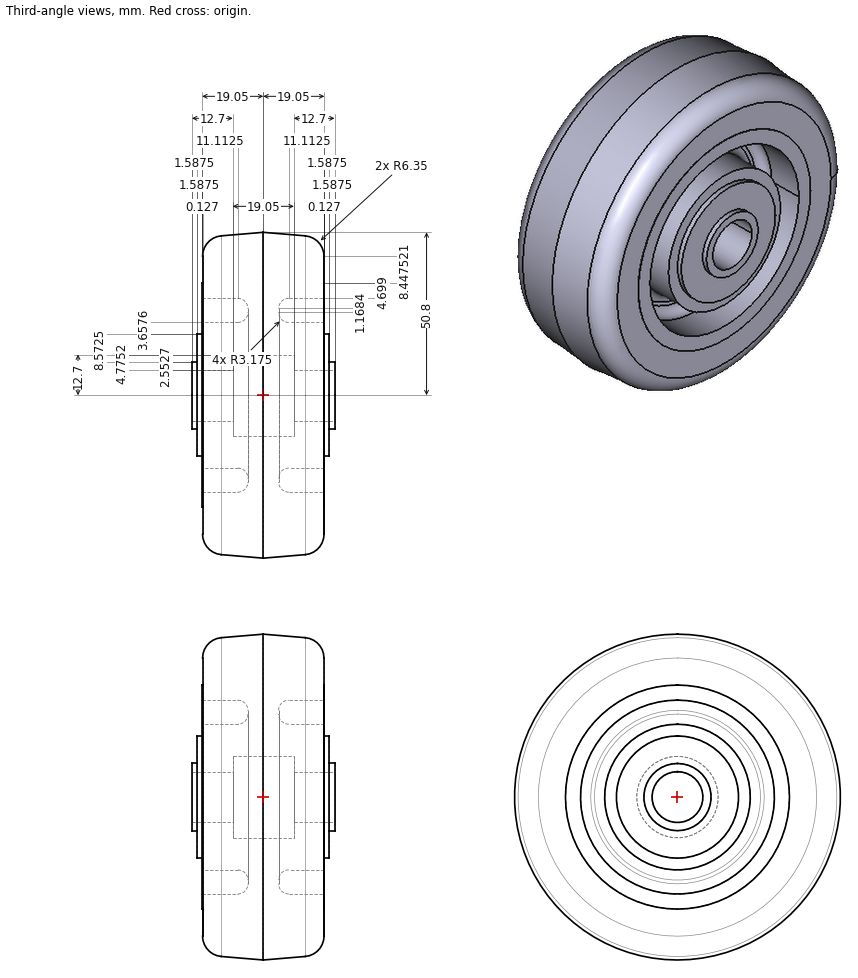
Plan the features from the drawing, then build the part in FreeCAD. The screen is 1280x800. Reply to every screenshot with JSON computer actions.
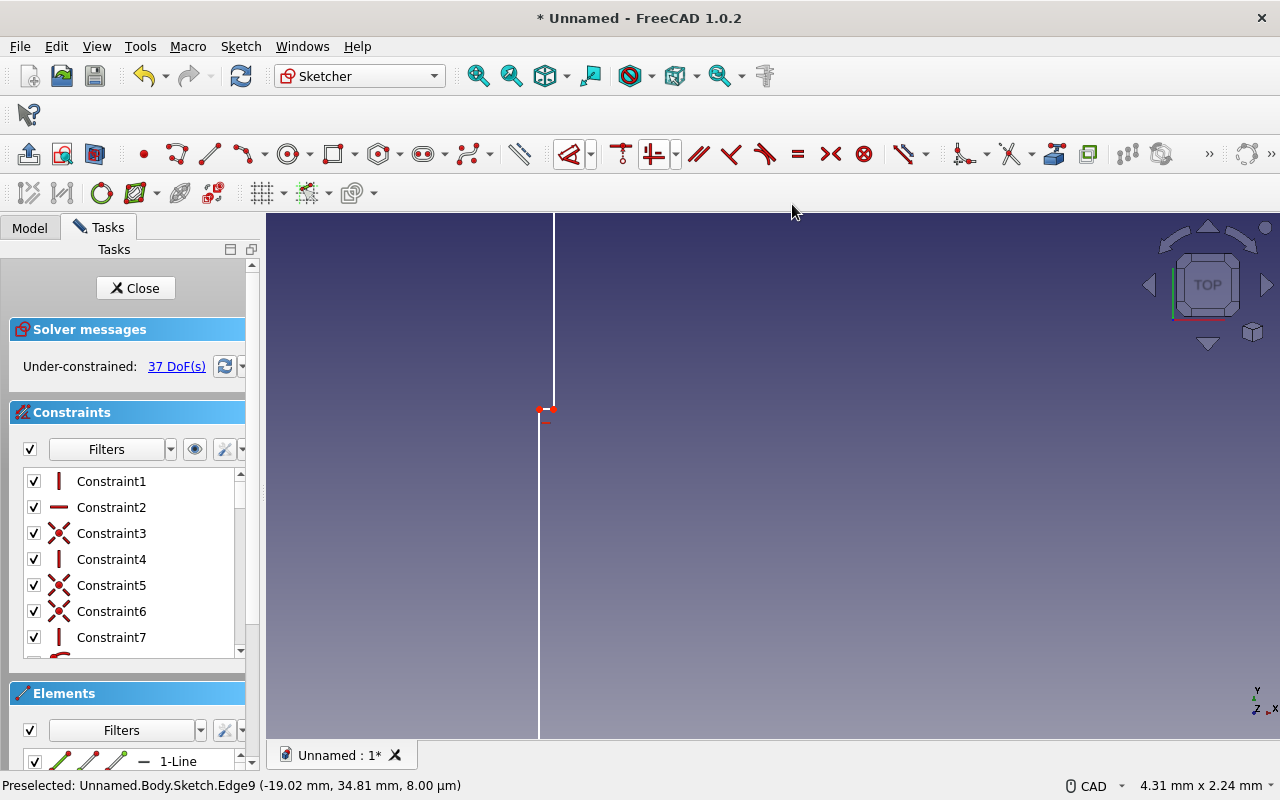
{"action": "scroll", "coordinate": [556, 402], "scroll_direction": "down", "scroll_amount": 17}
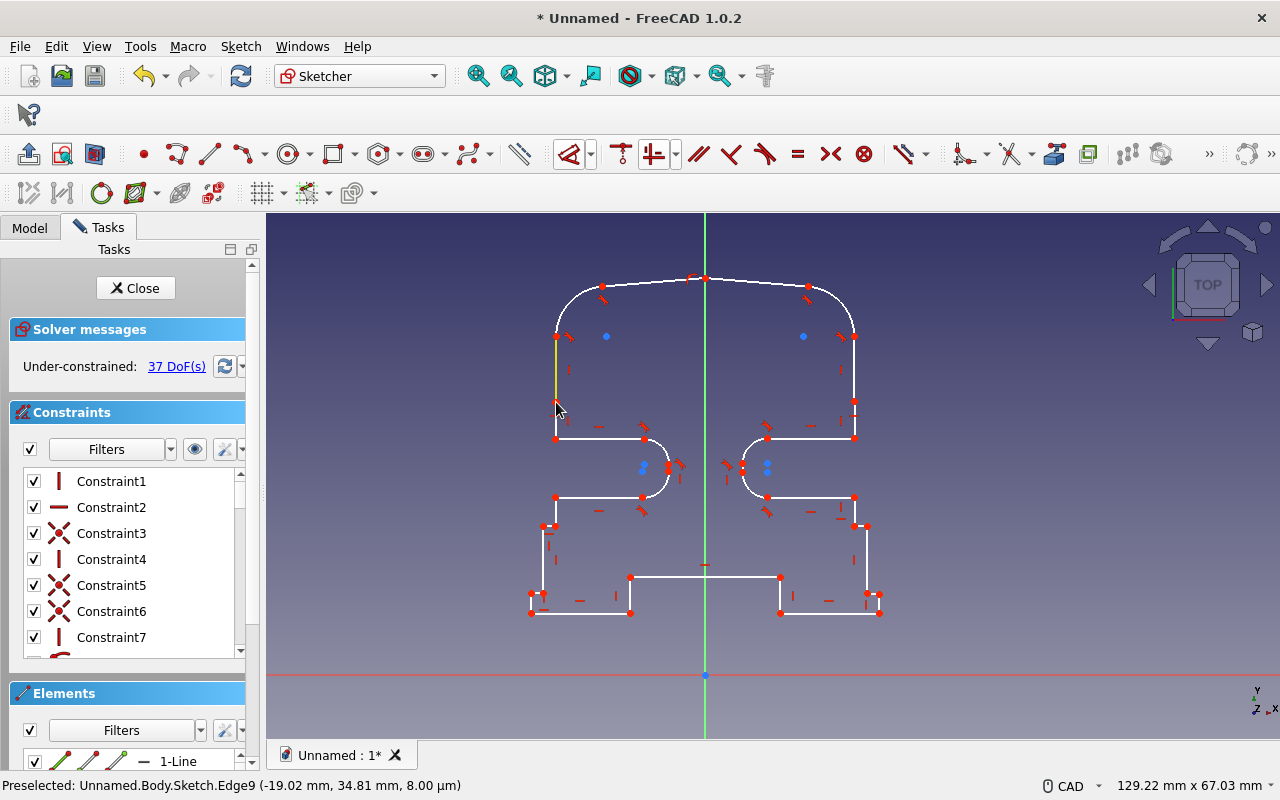
{"action": "scroll", "coordinate": [876, 594], "scroll_direction": "up", "scroll_amount": 7}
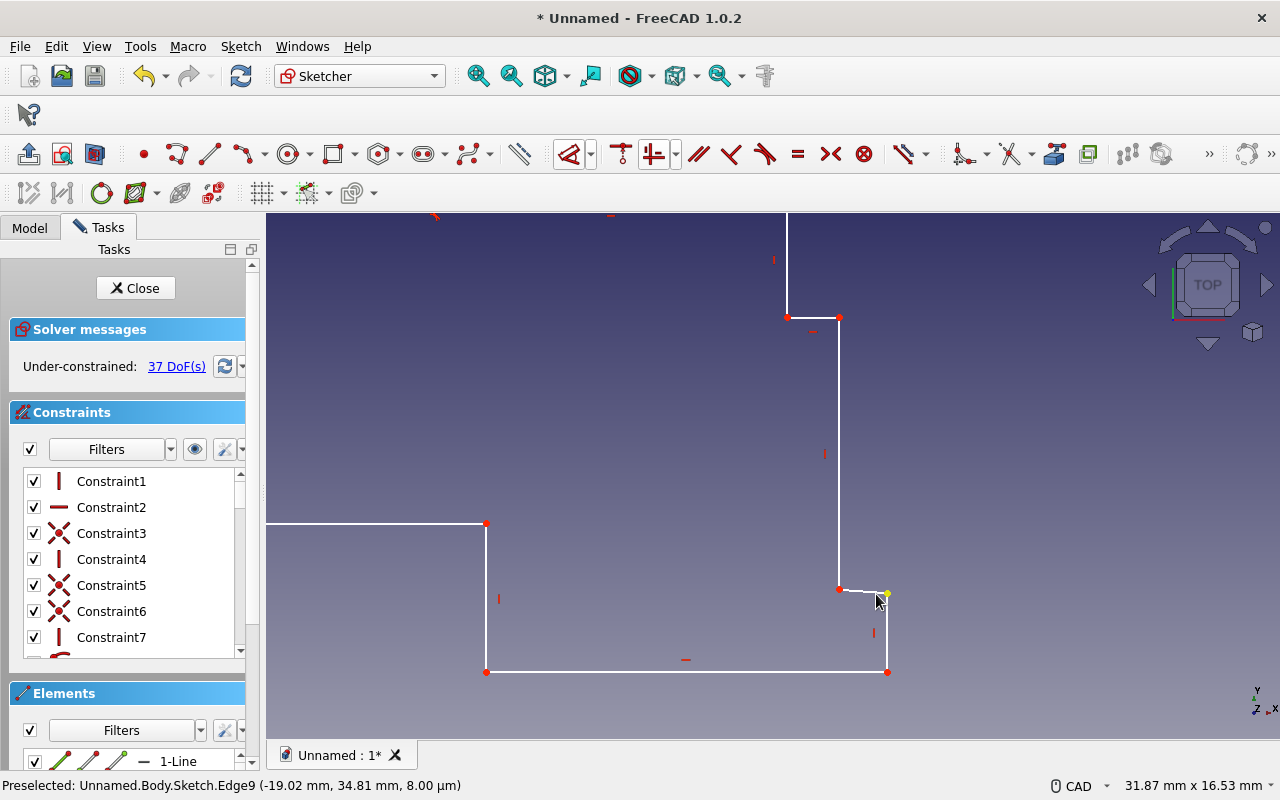
{"action": "left_click", "coordinate": [873, 592]}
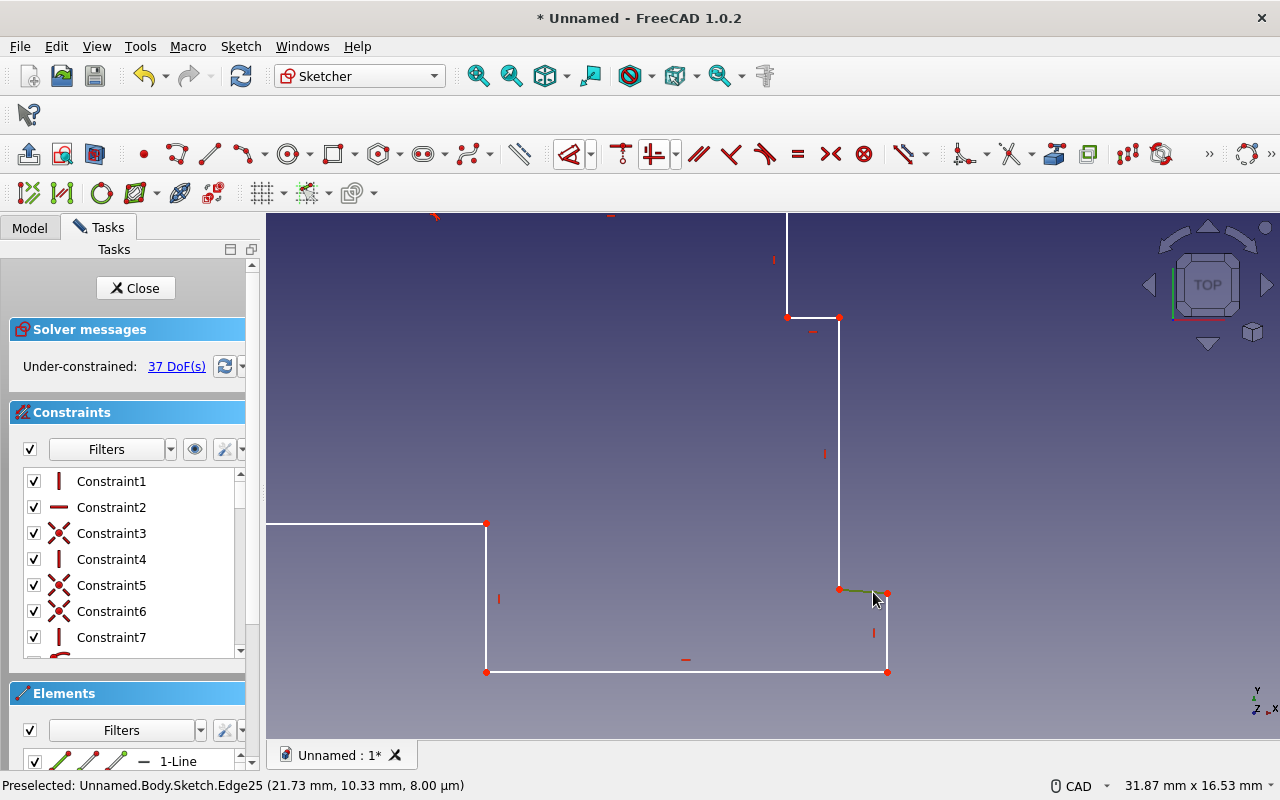
{"action": "left_click", "coordinate": [676, 154]}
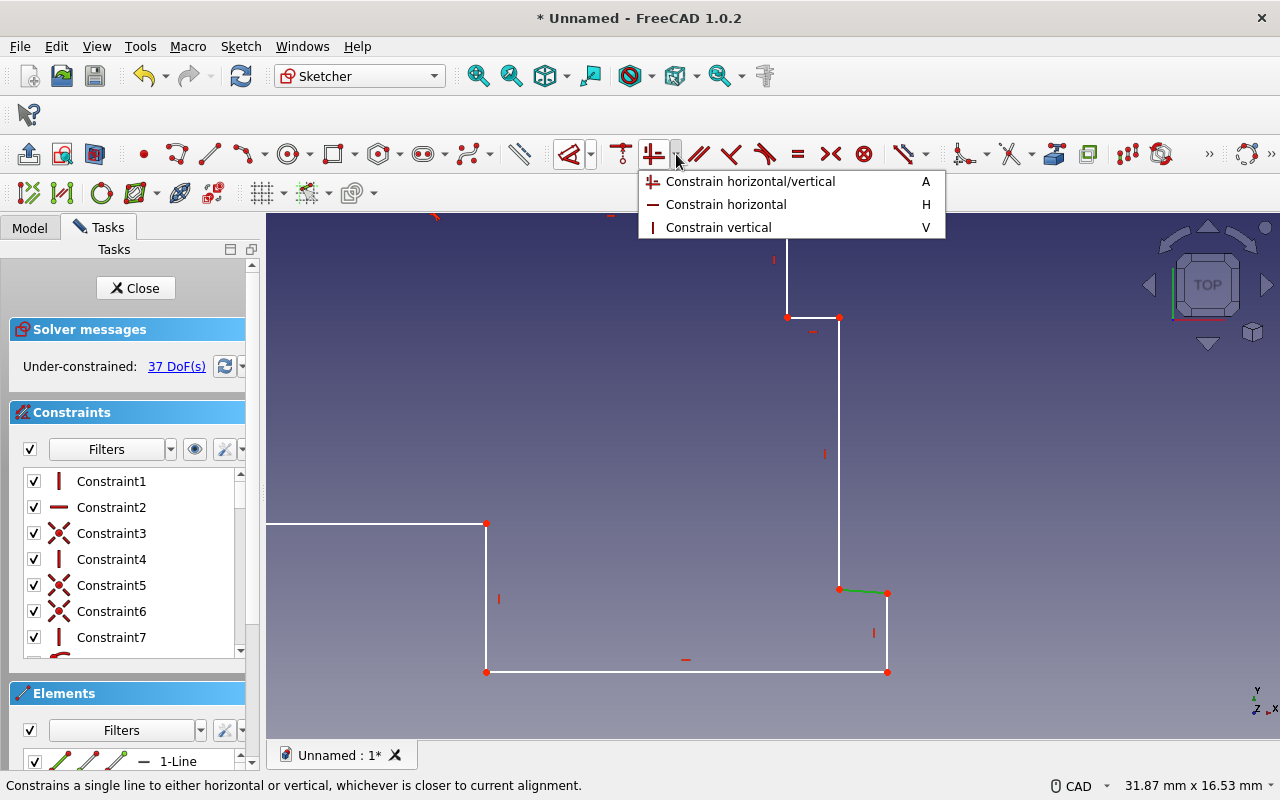
{"action": "left_click", "coordinate": [792, 204]}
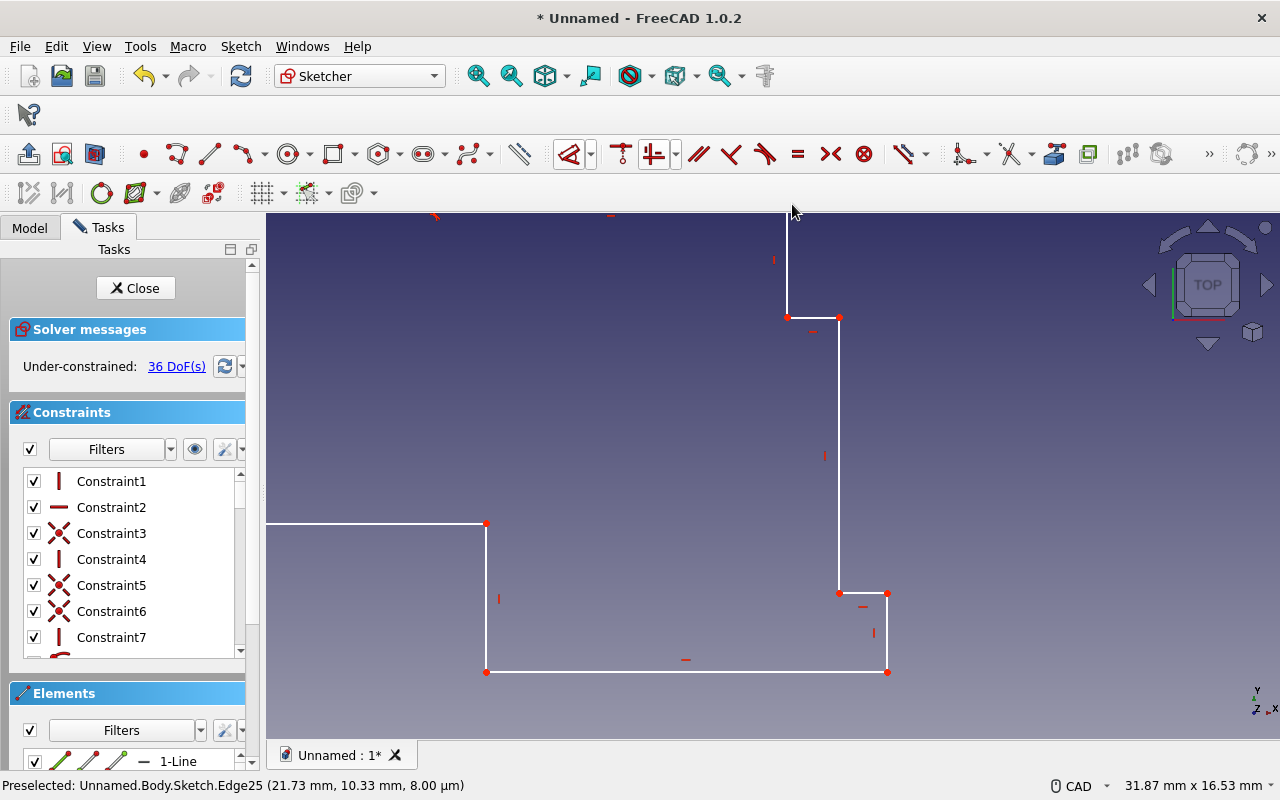
{"action": "scroll", "coordinate": [837, 568], "scroll_direction": "down", "scroll_amount": 8}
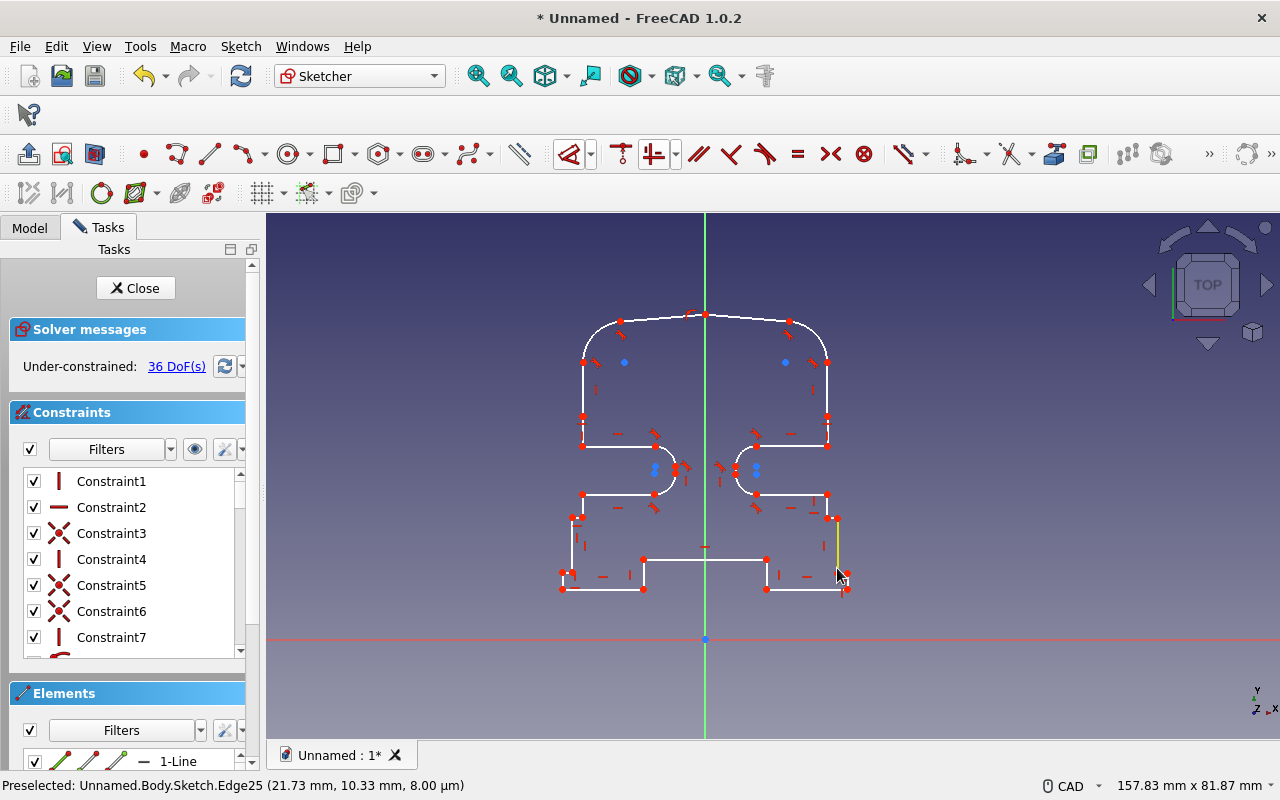
{"action": "left_click", "coordinate": [823, 345]}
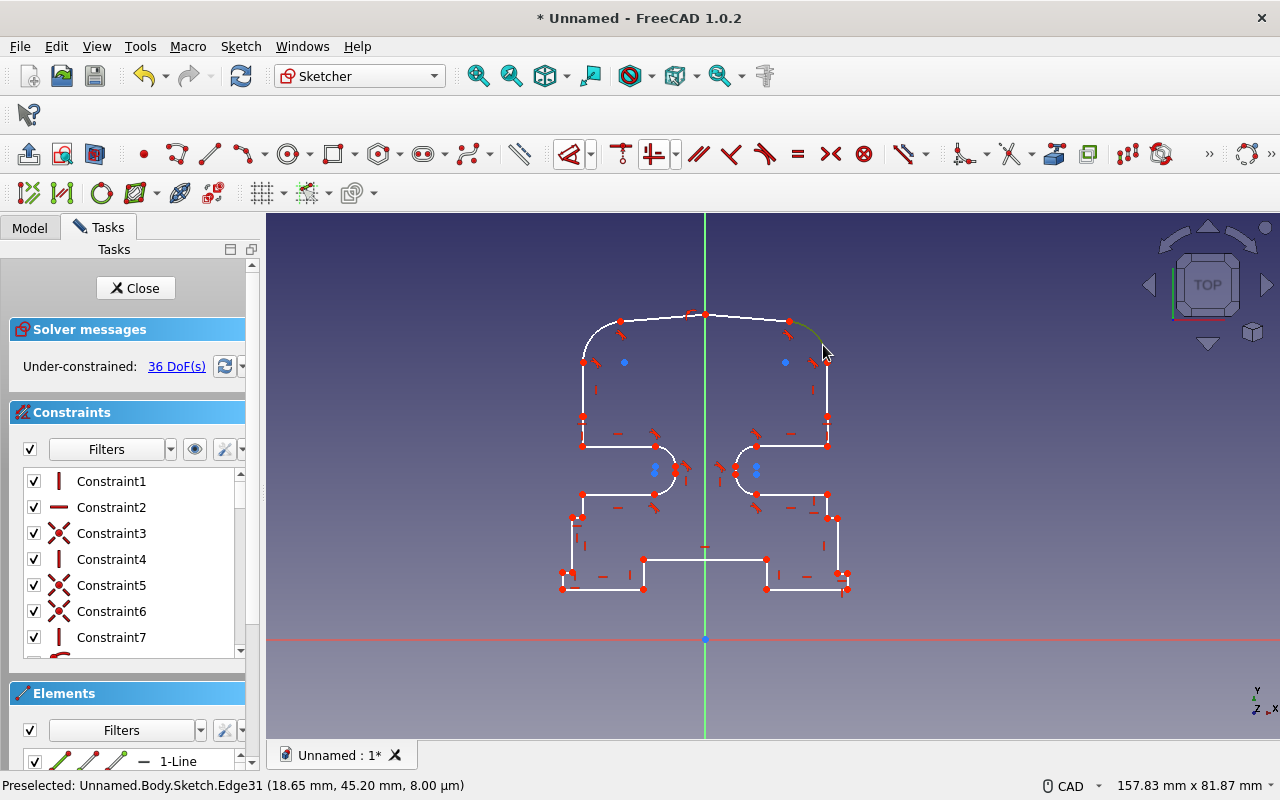
{"action": "left_click", "coordinate": [603, 327]}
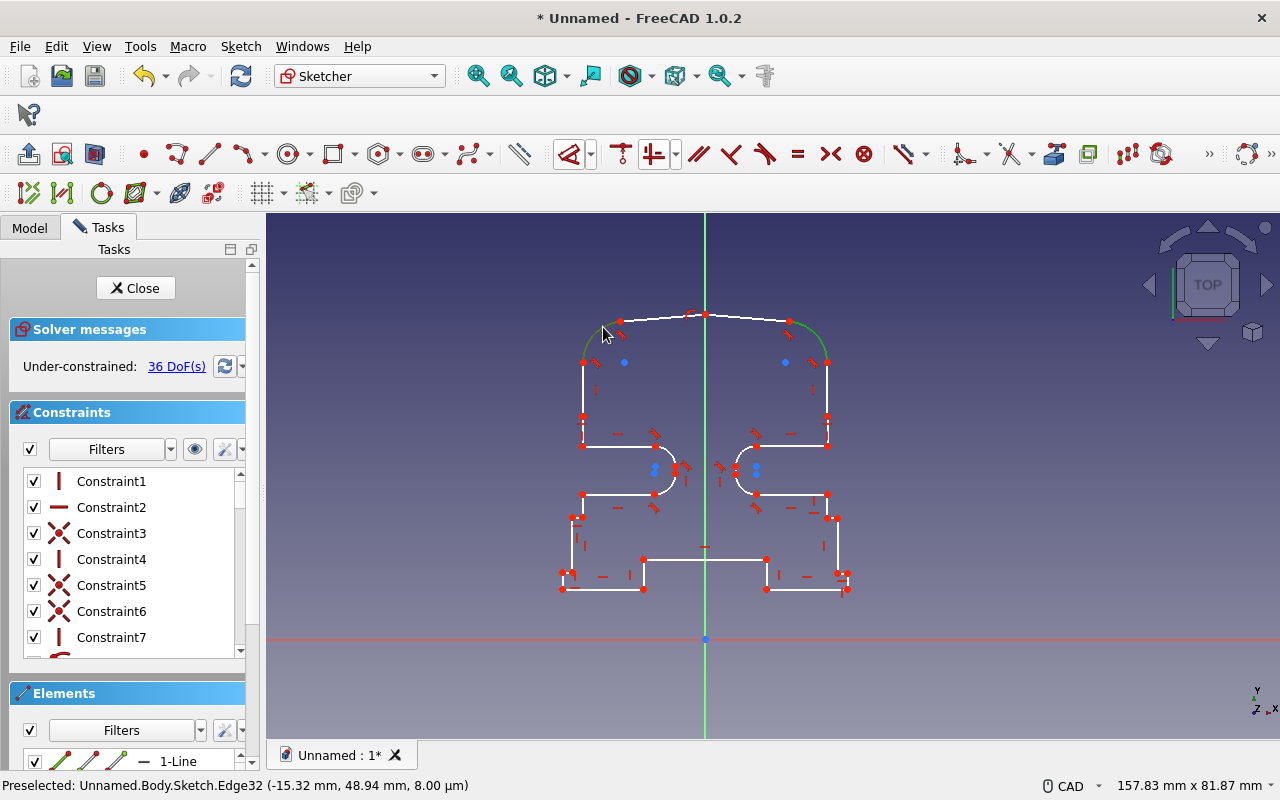
{"action": "left_click", "coordinate": [798, 154]}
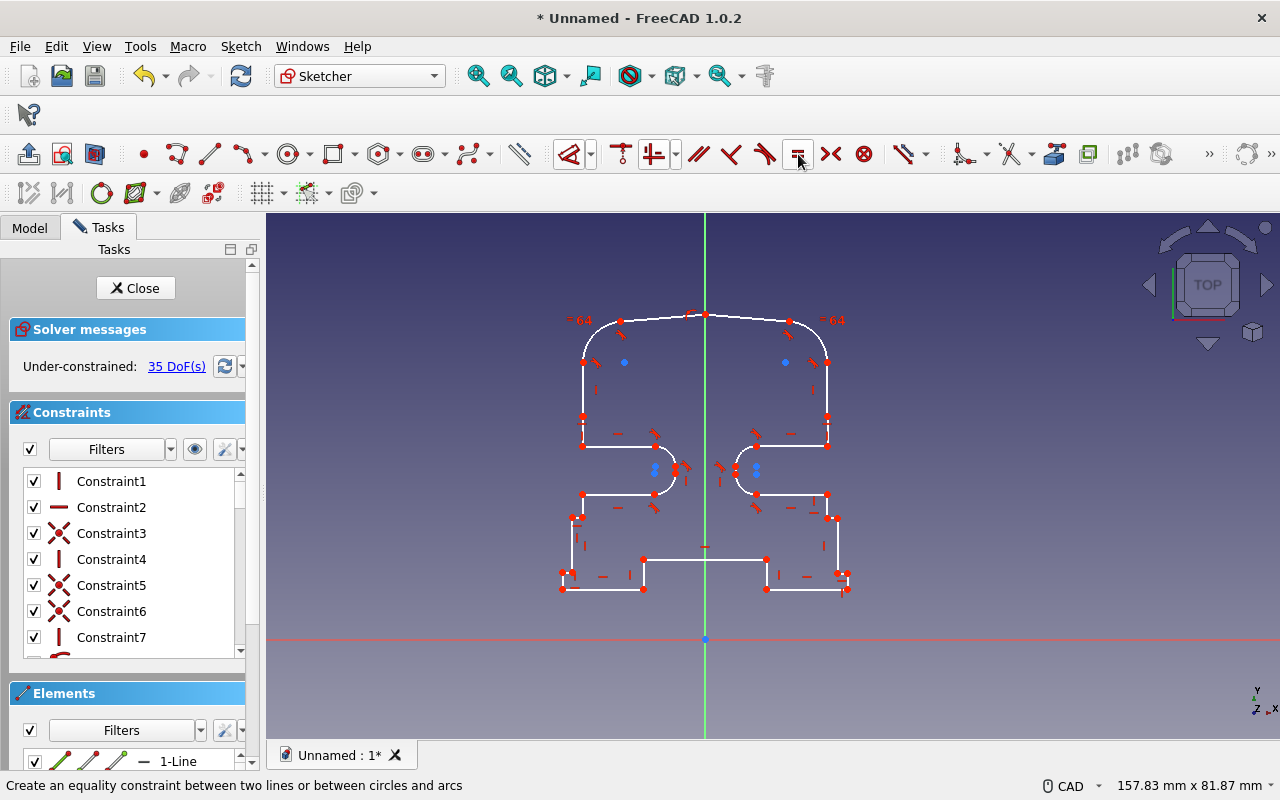
{"action": "scroll", "coordinate": [747, 448], "scroll_direction": "up", "scroll_amount": 2}